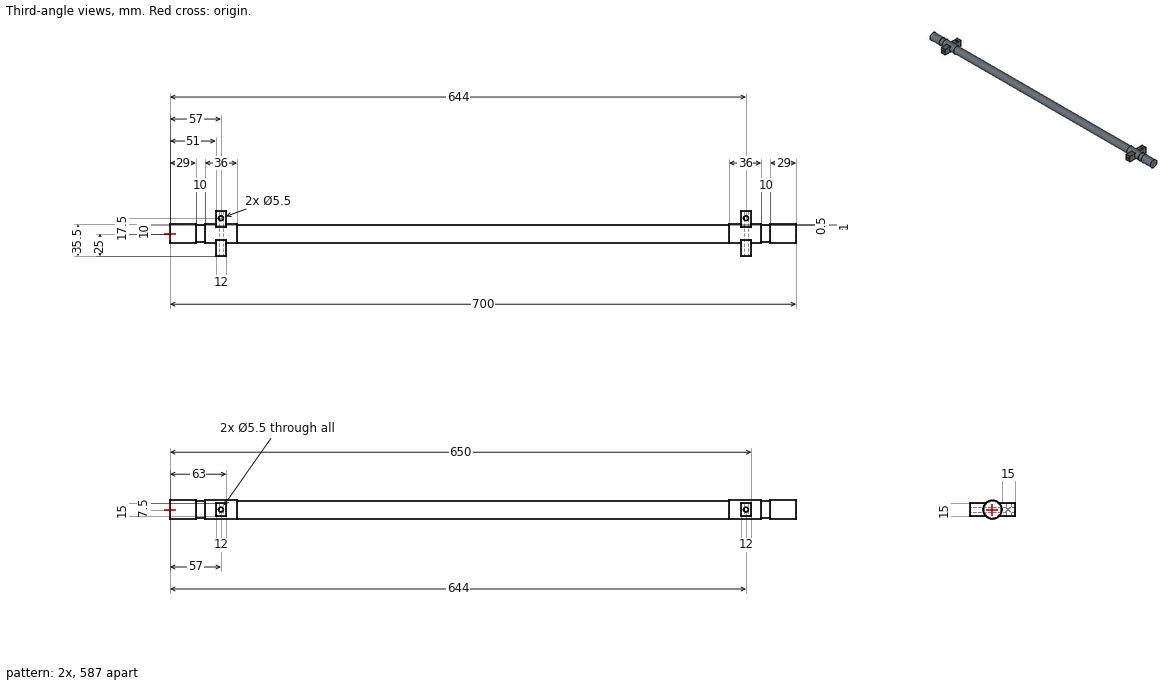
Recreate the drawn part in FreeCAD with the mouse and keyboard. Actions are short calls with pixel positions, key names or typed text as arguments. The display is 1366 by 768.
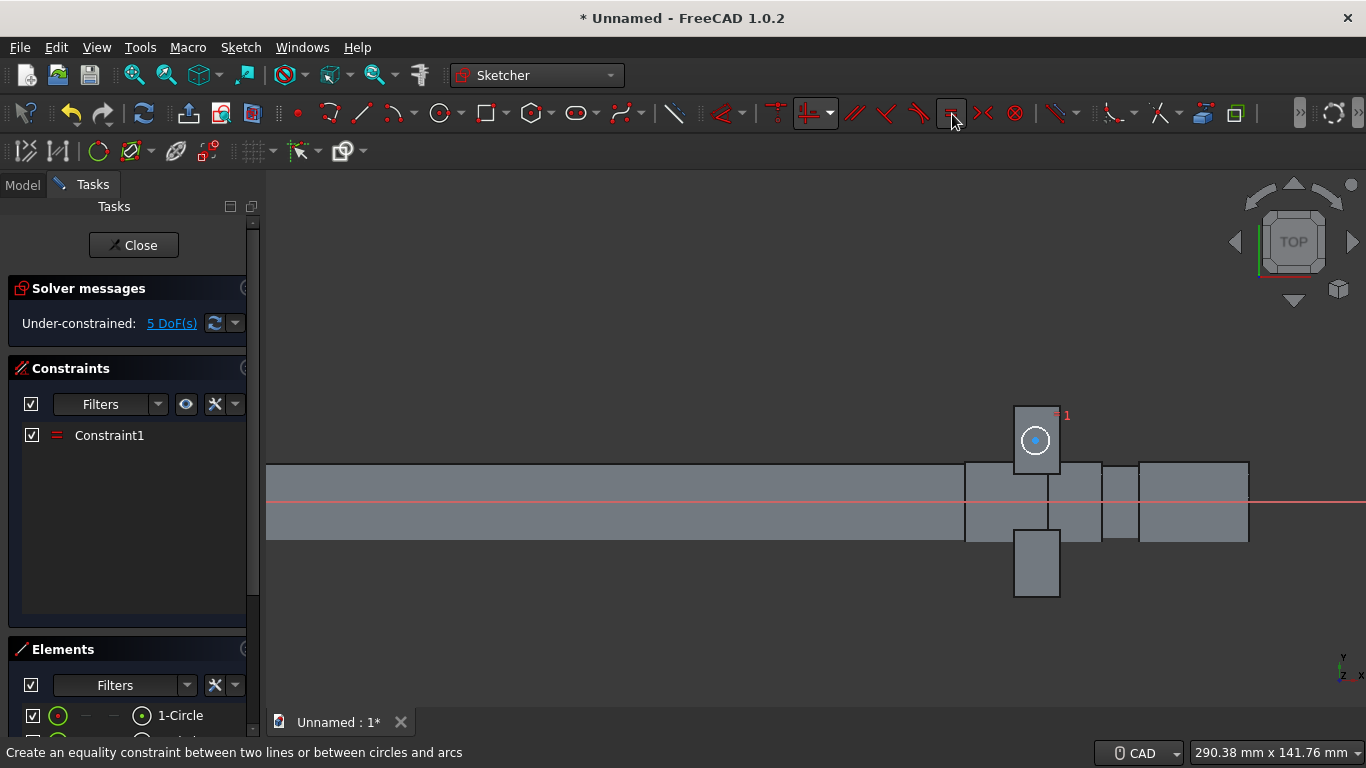
scroll(1050, 430, down, 7)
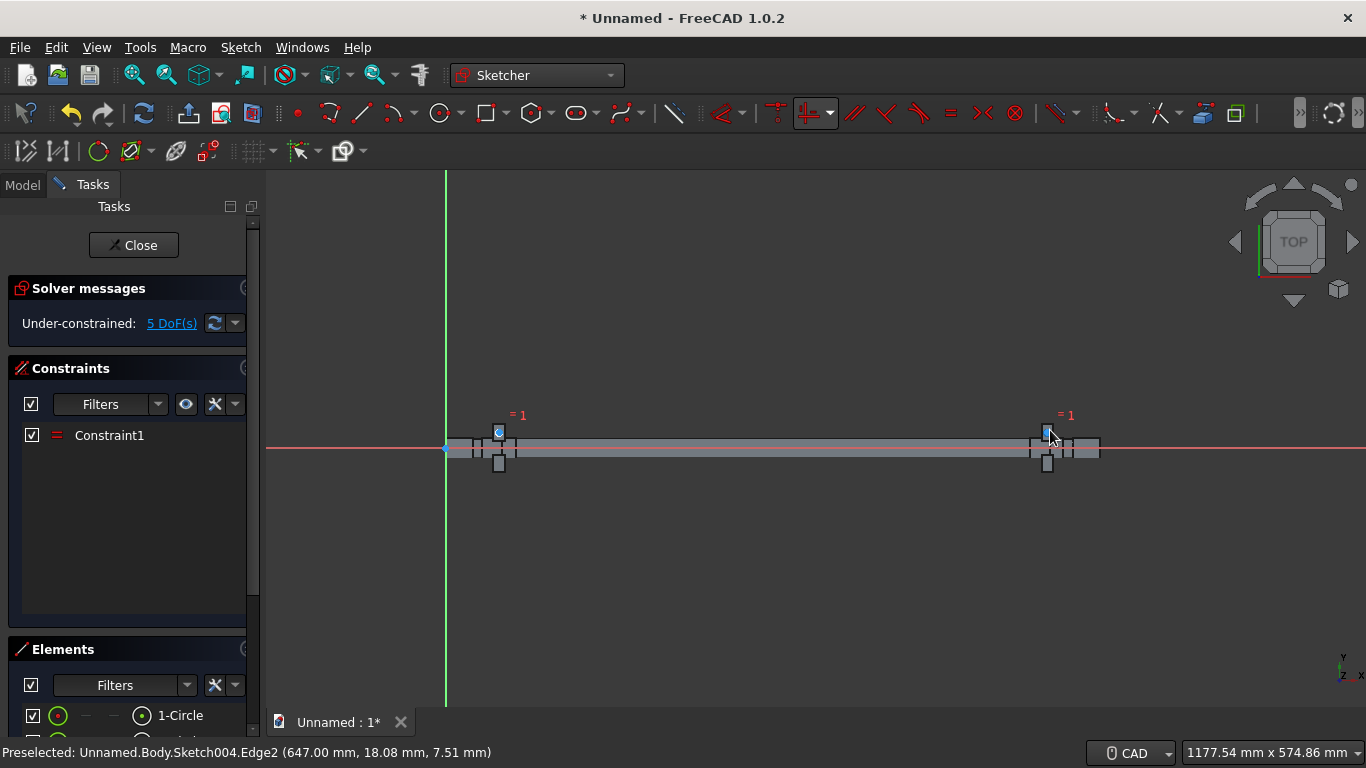
click(499, 433)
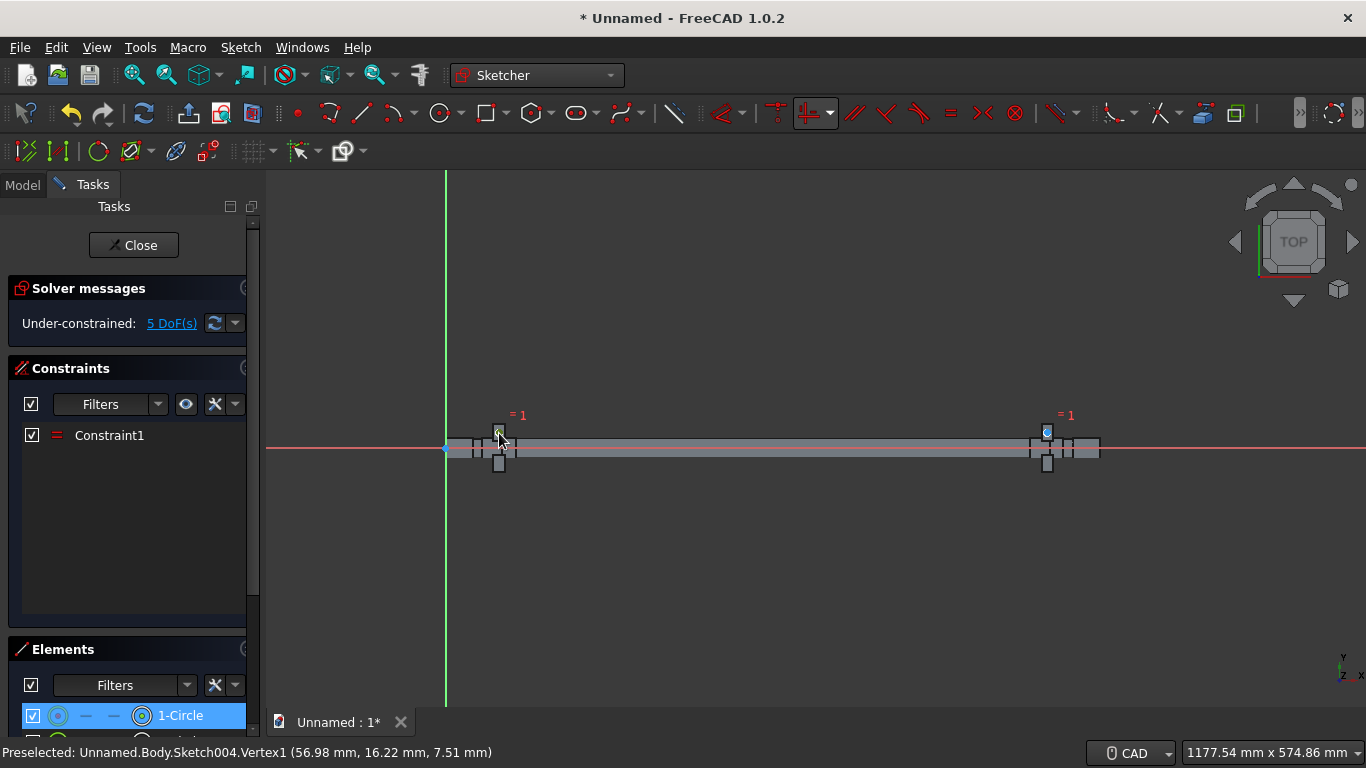
click(1047, 433)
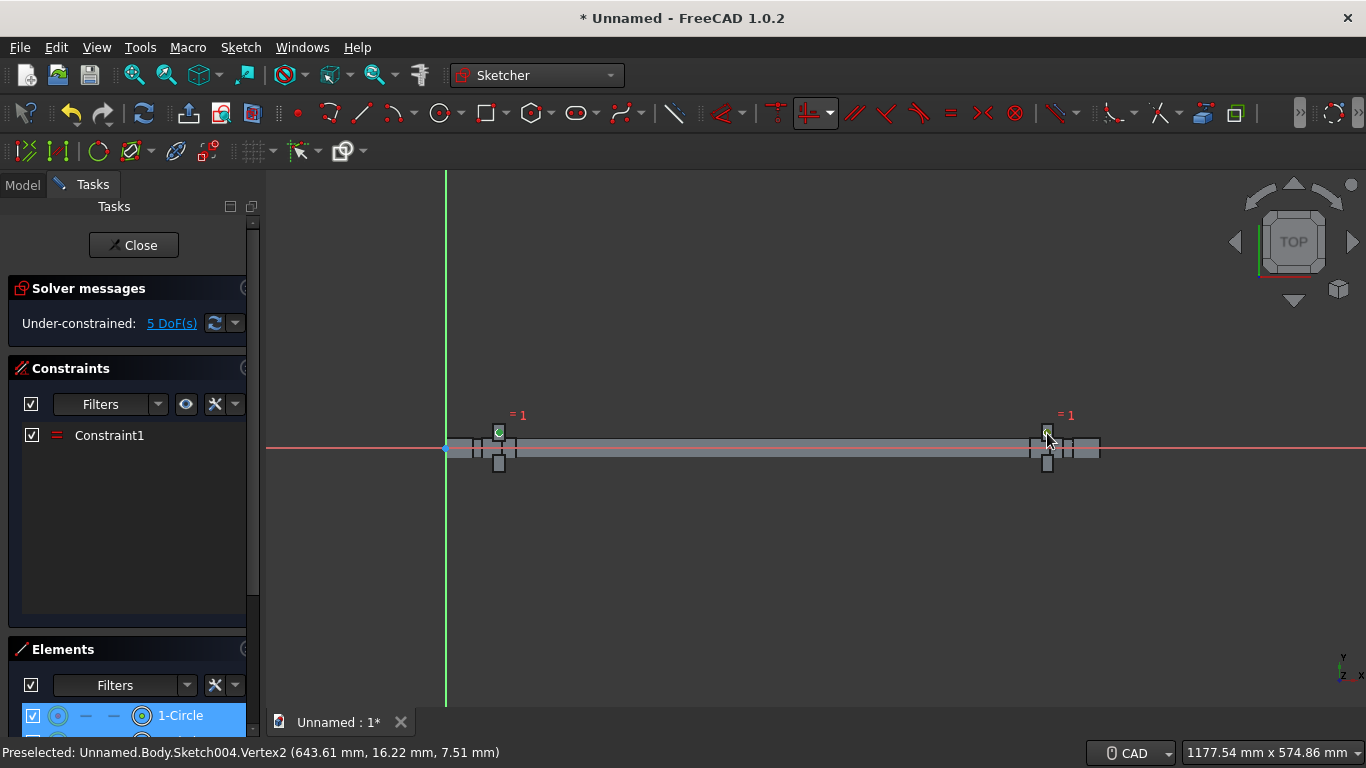
key(h)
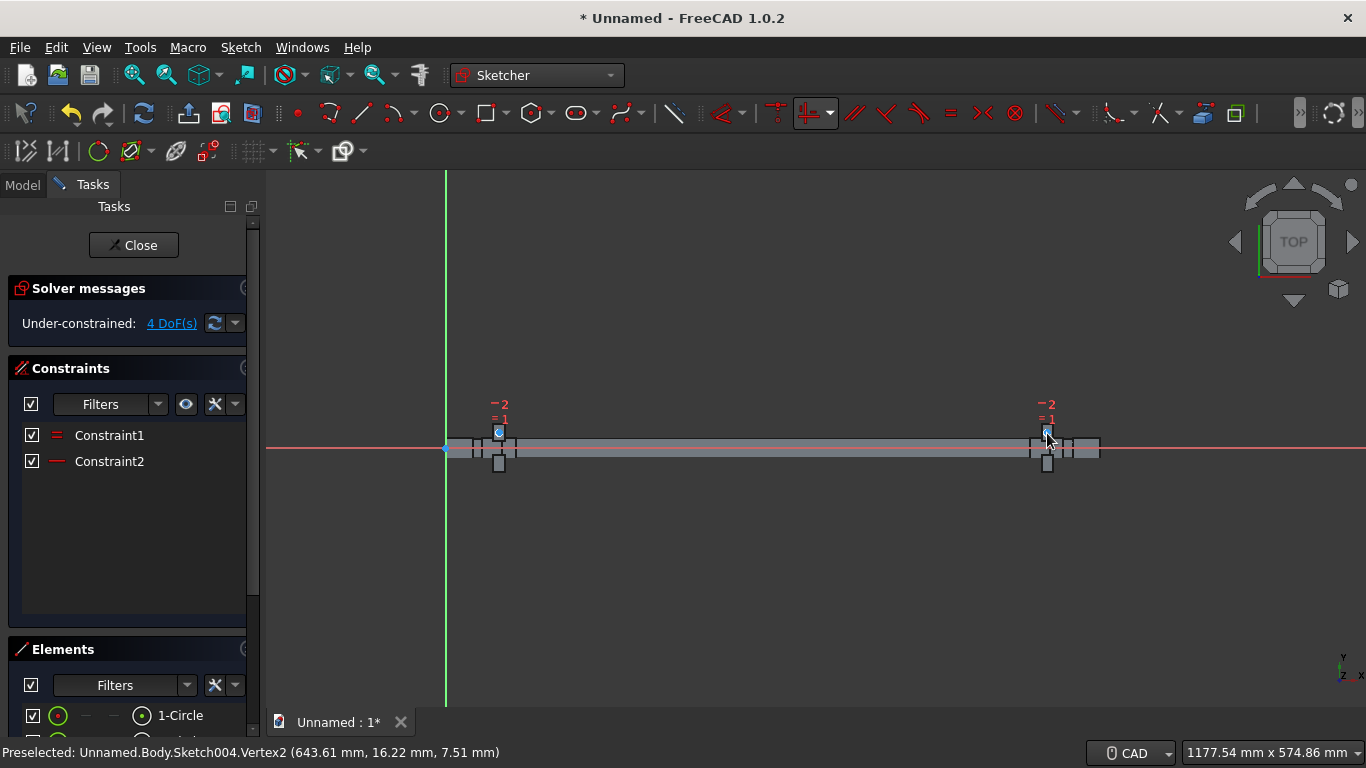
key(d)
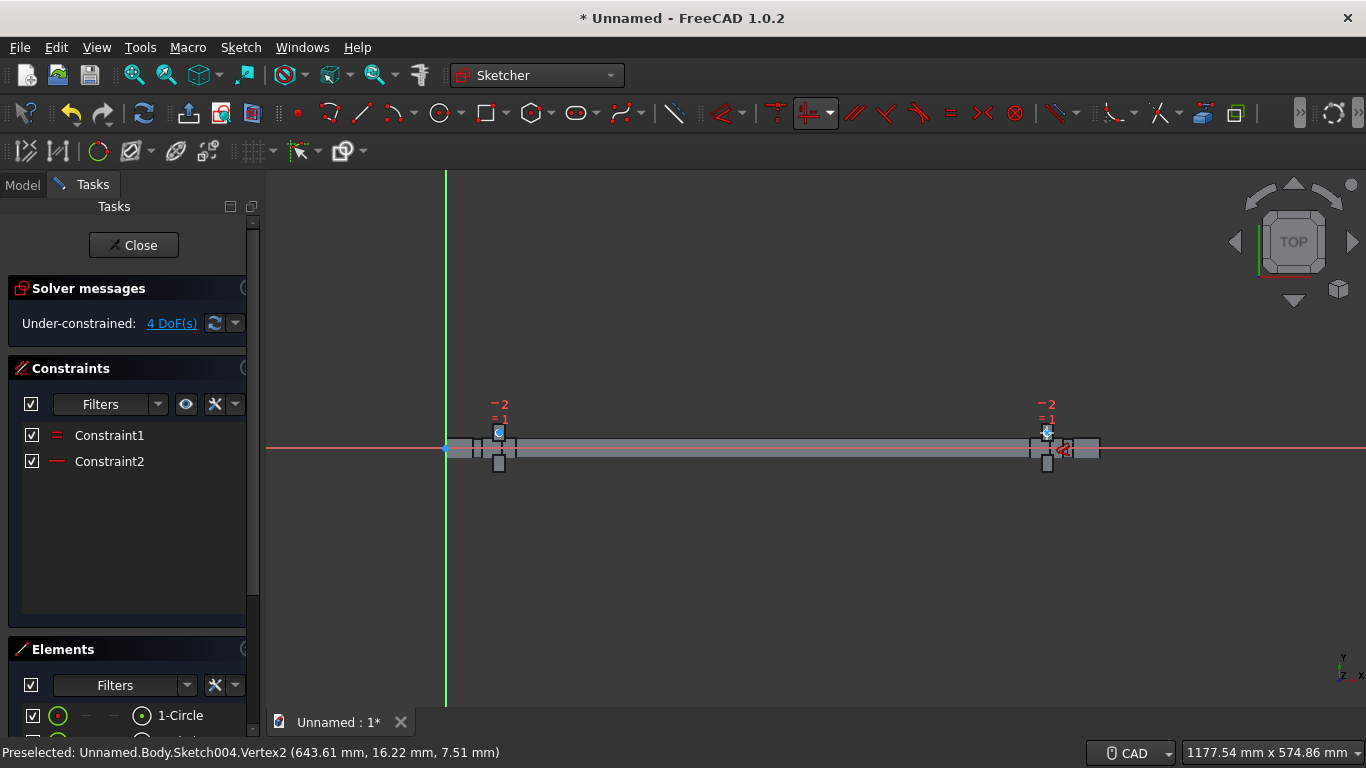
scroll(497, 431, up, 11)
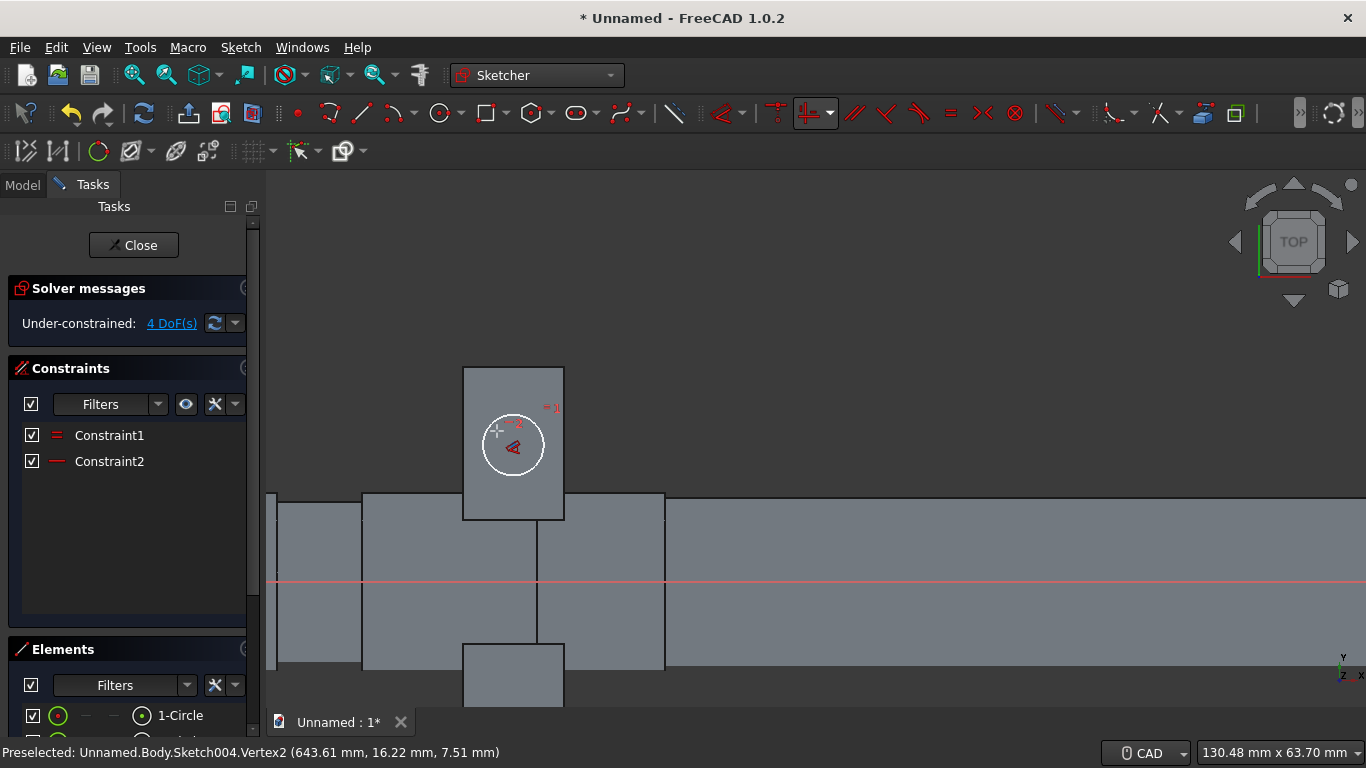
click(492, 424)
click(469, 401)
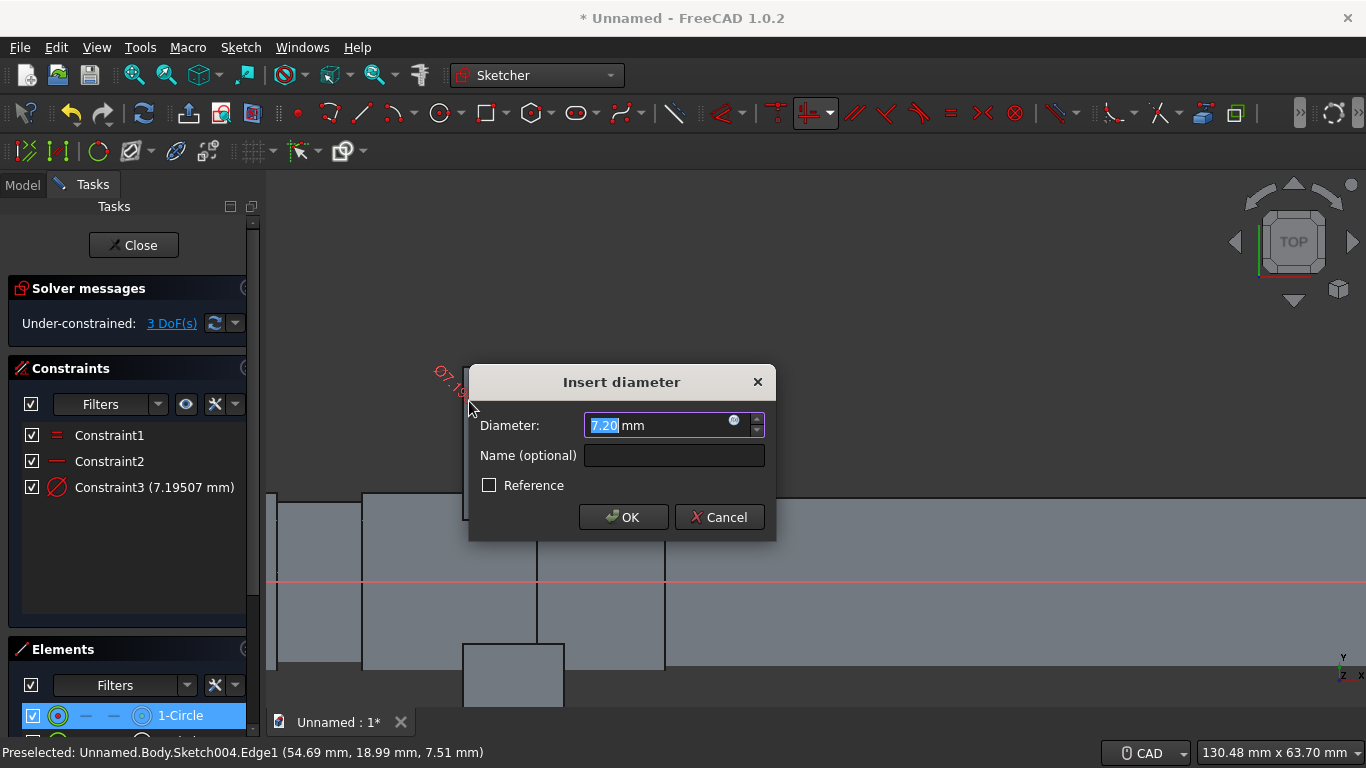
text(5.5)
key(Return)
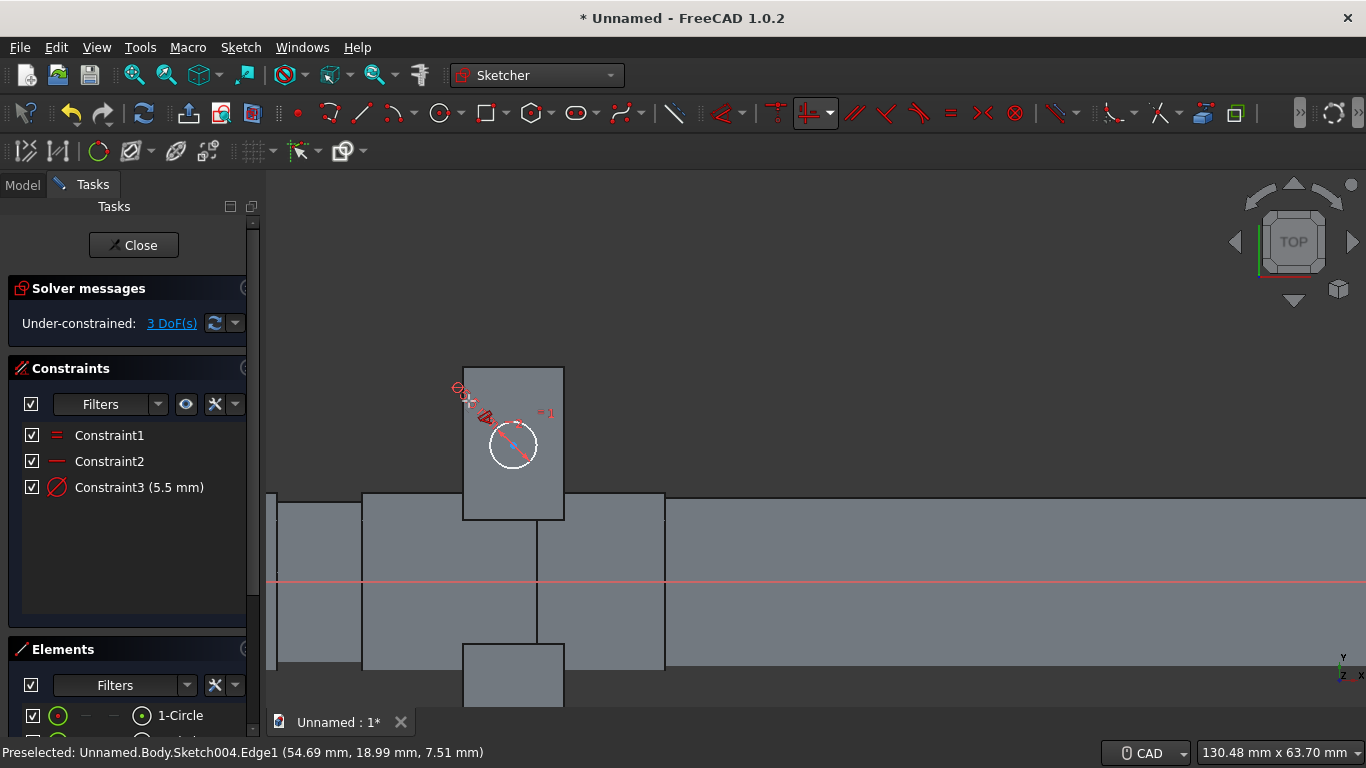
scroll(497, 431, down, 11)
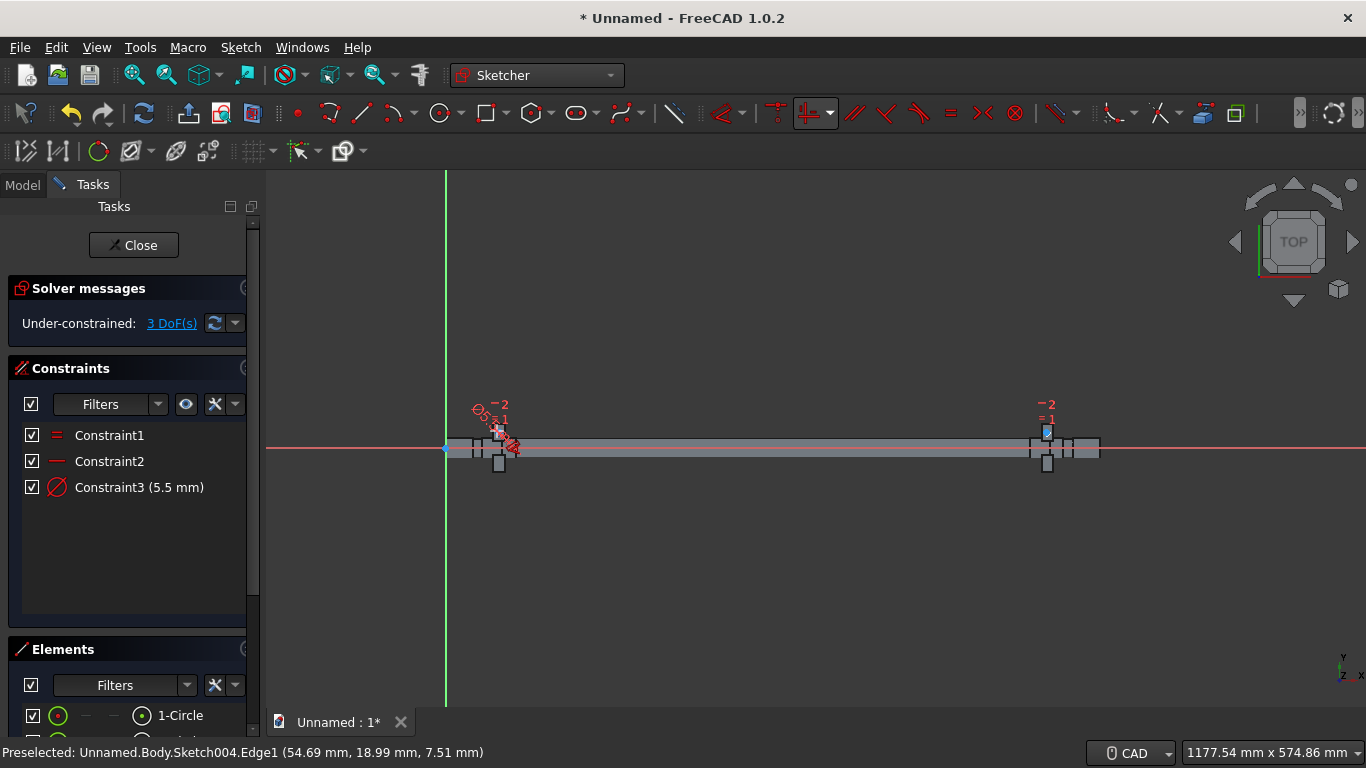
click(499, 433)
click(472, 482)